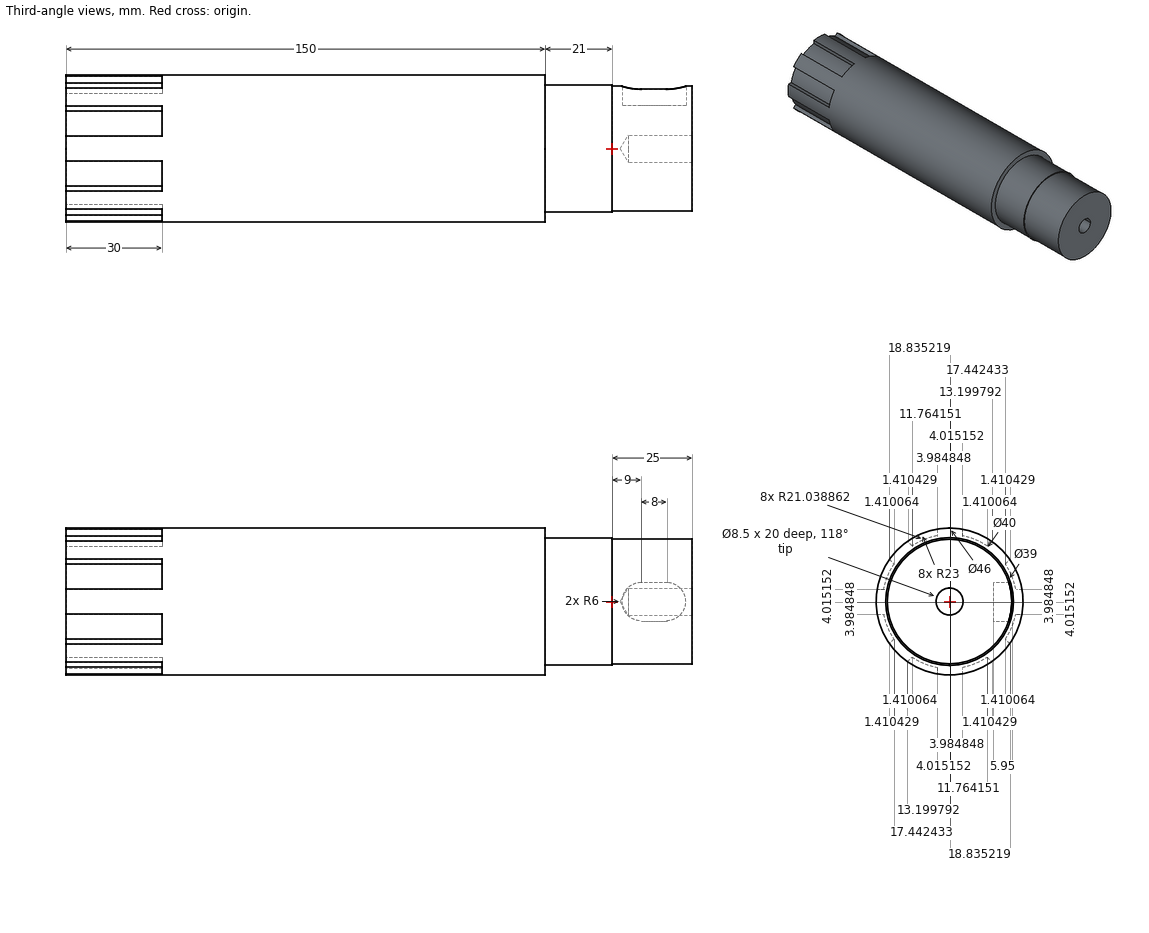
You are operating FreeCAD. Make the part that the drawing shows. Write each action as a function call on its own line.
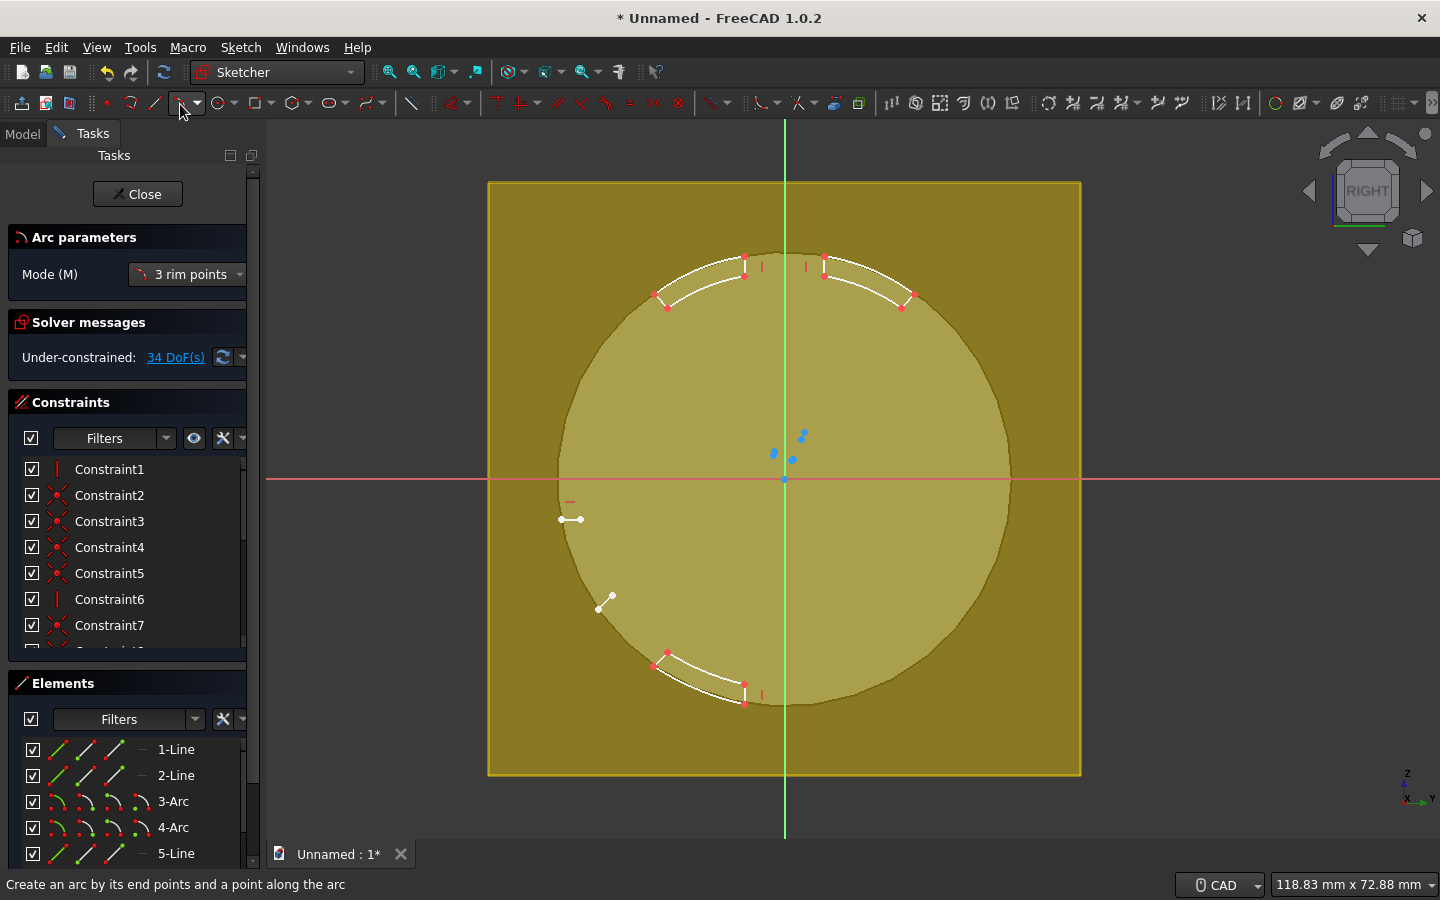
scroll(598, 609, up, 3)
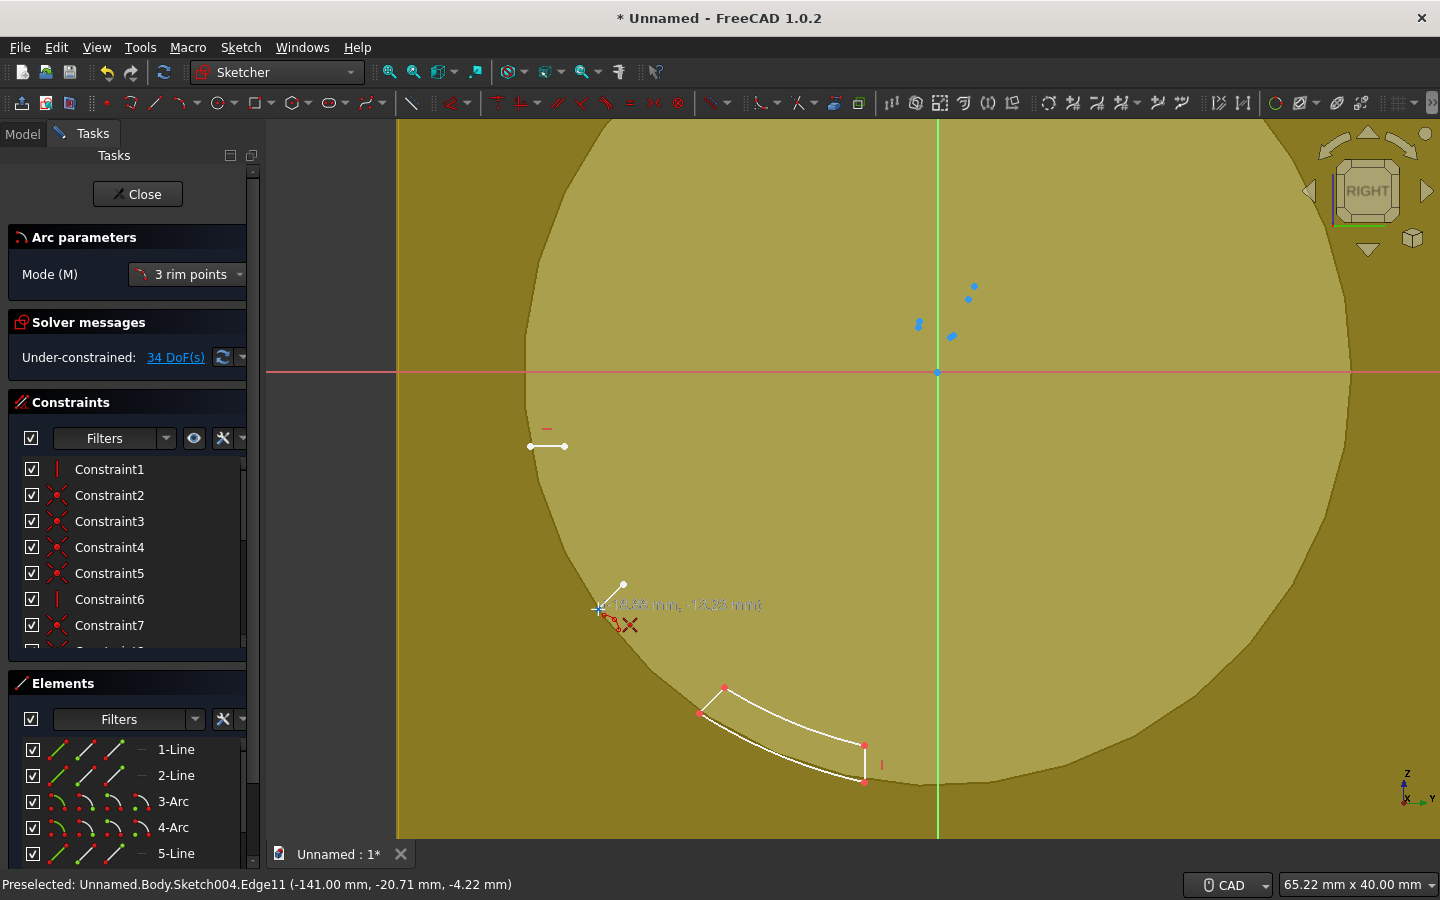
click(598, 610)
click(530, 446)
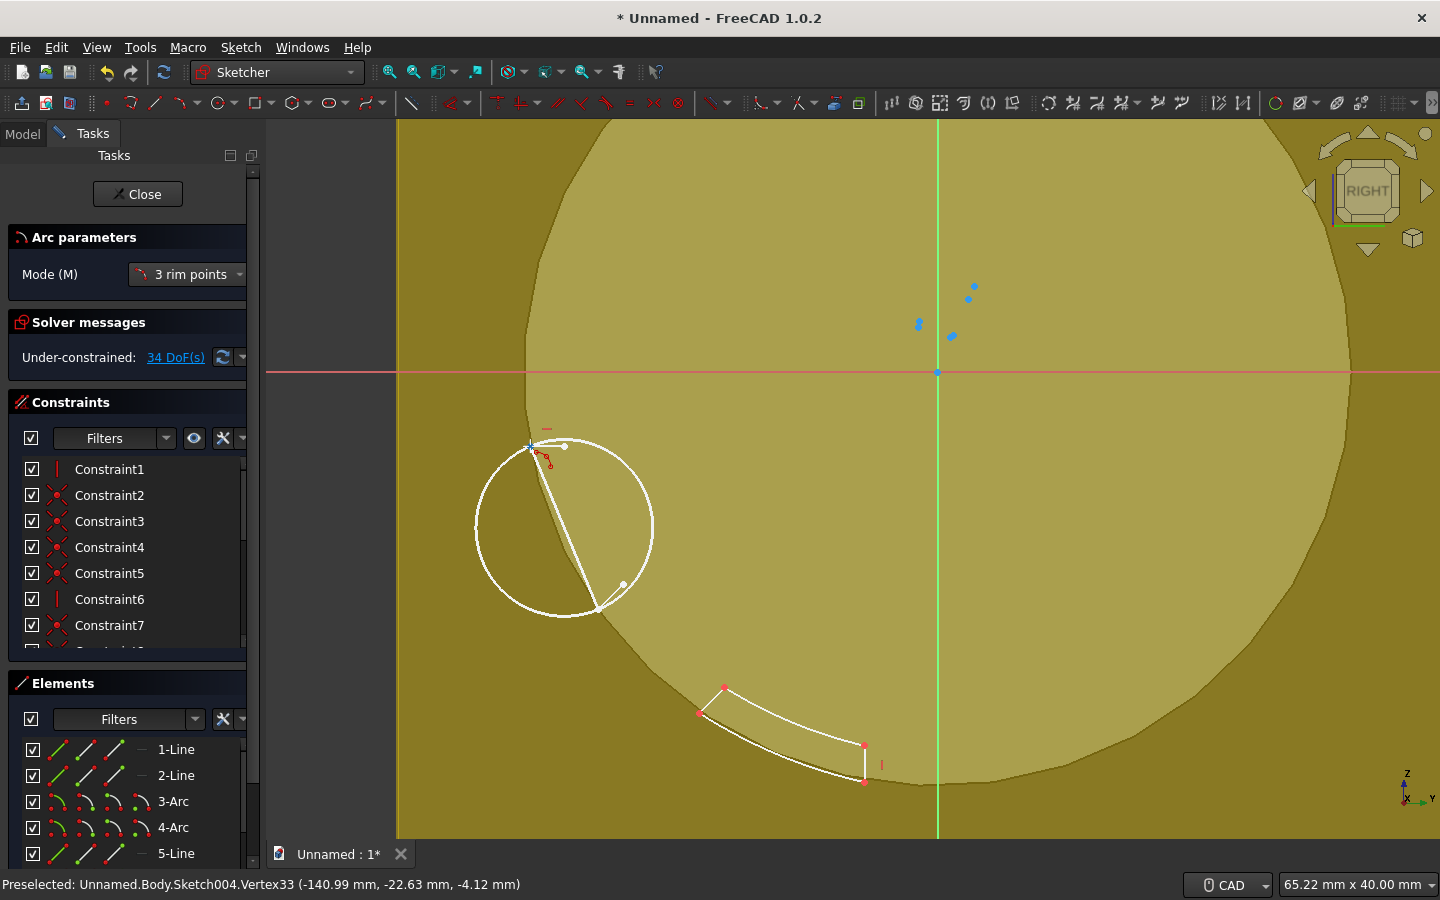
scroll(555, 530, up, 3)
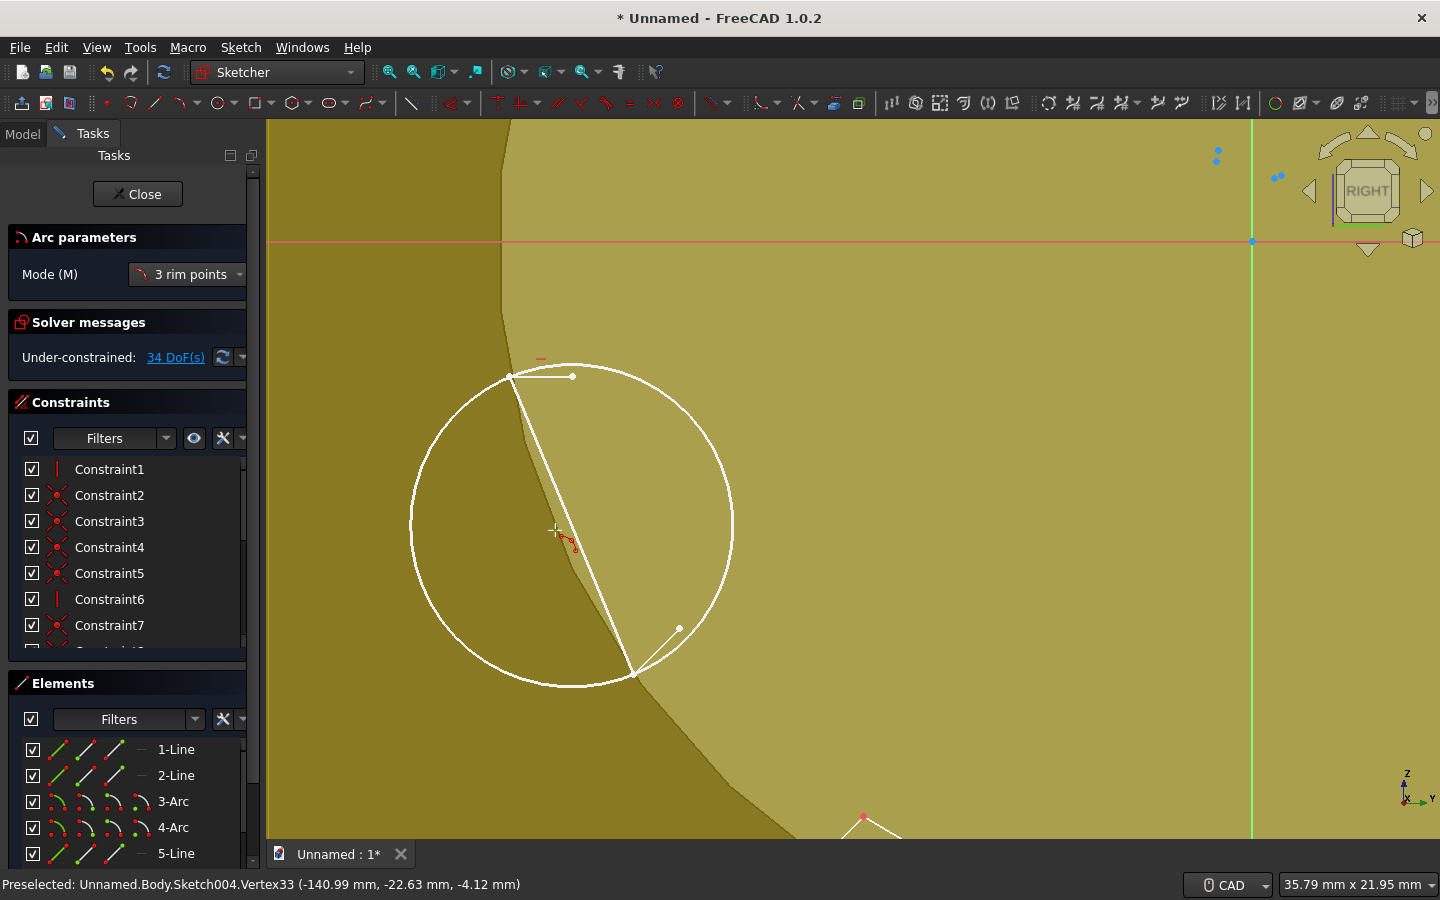
click(555, 530)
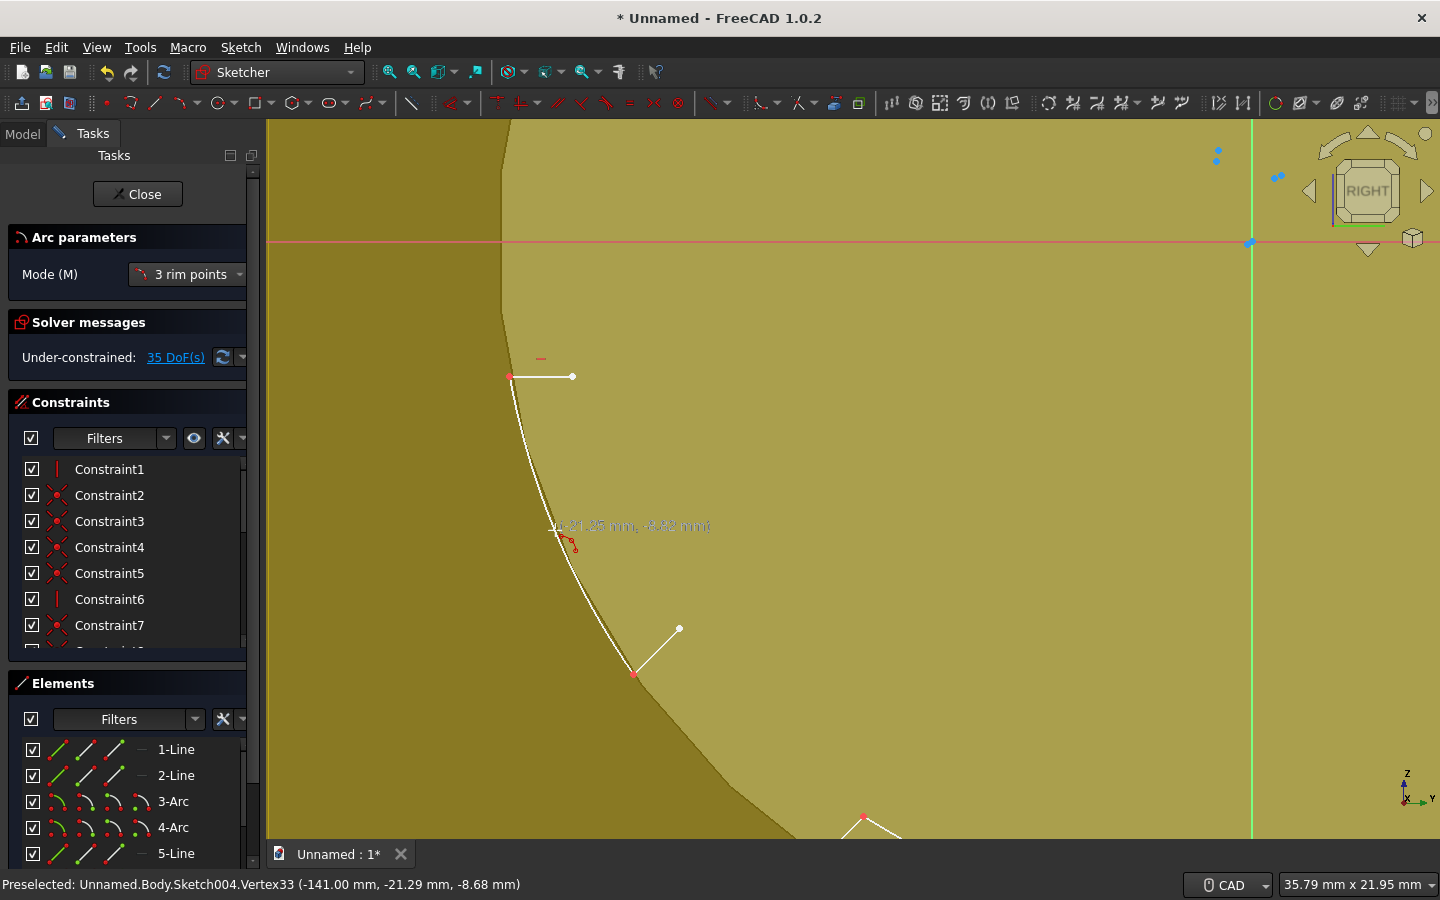
click(573, 377)
click(680, 629)
click(614, 505)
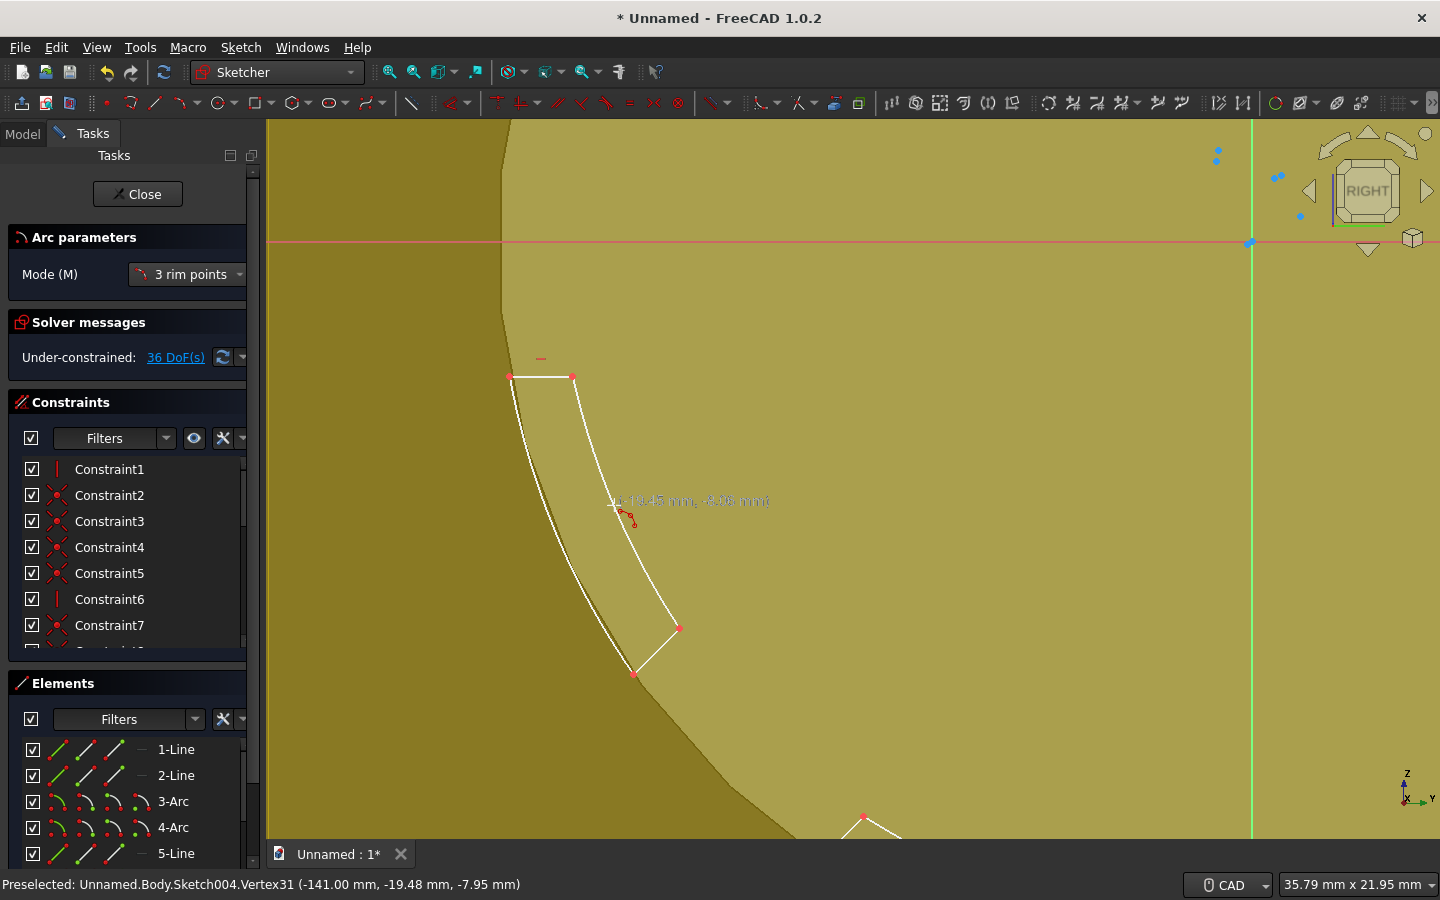
click(156, 104)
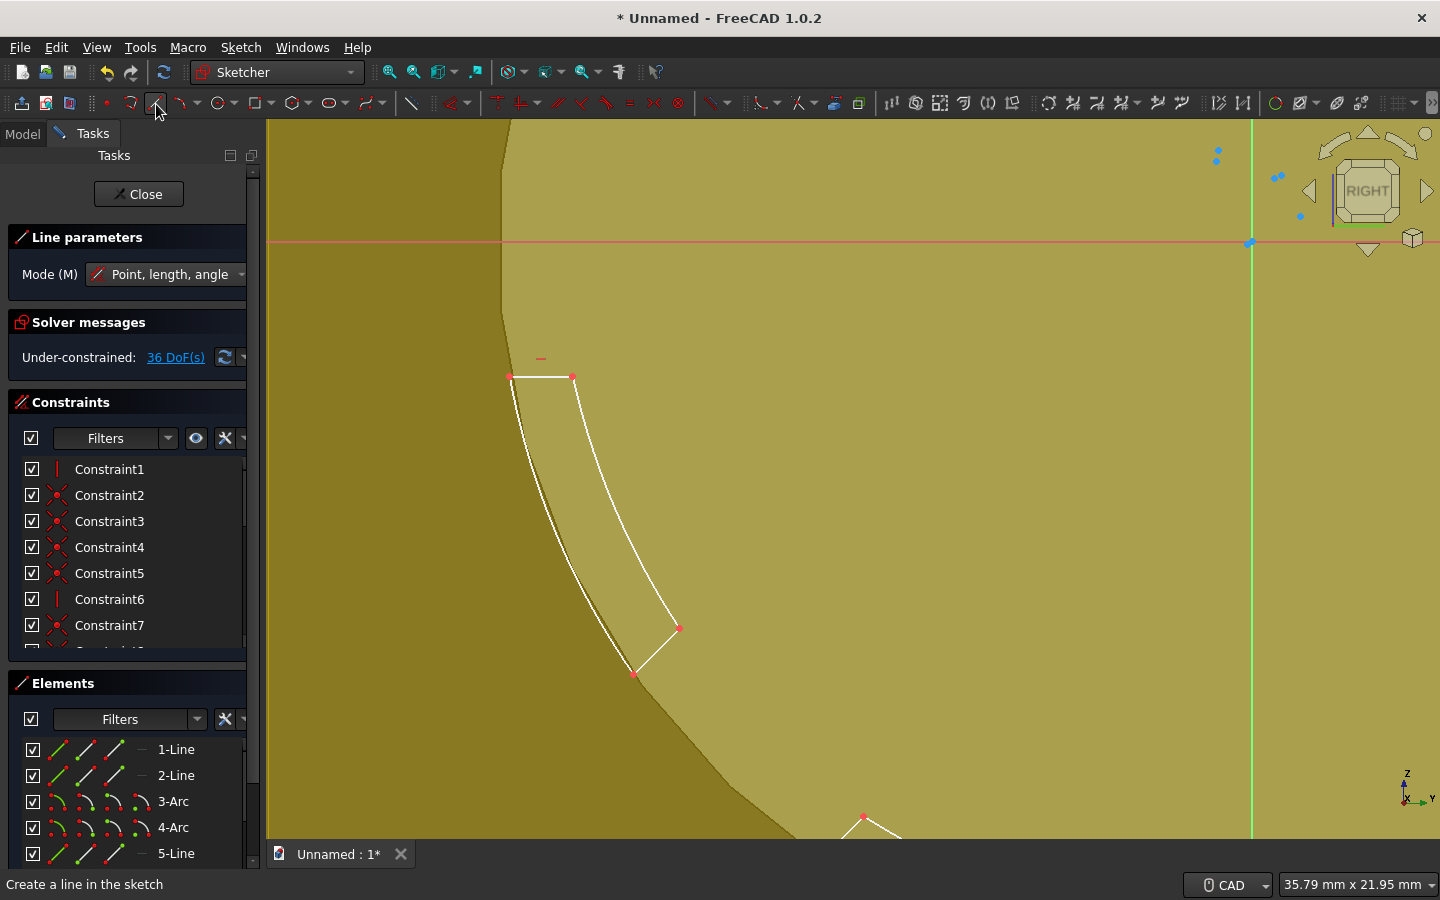
scroll(583, 581, down, 6)